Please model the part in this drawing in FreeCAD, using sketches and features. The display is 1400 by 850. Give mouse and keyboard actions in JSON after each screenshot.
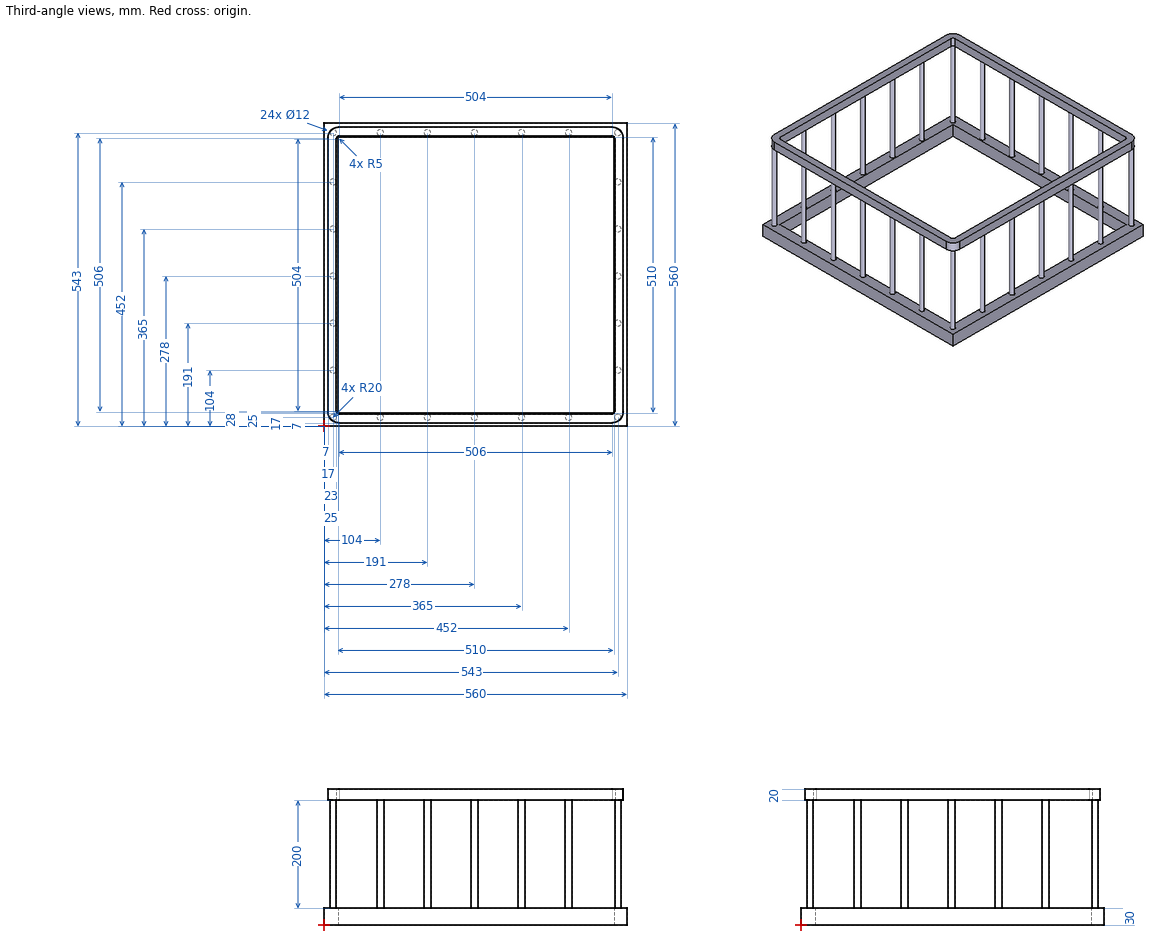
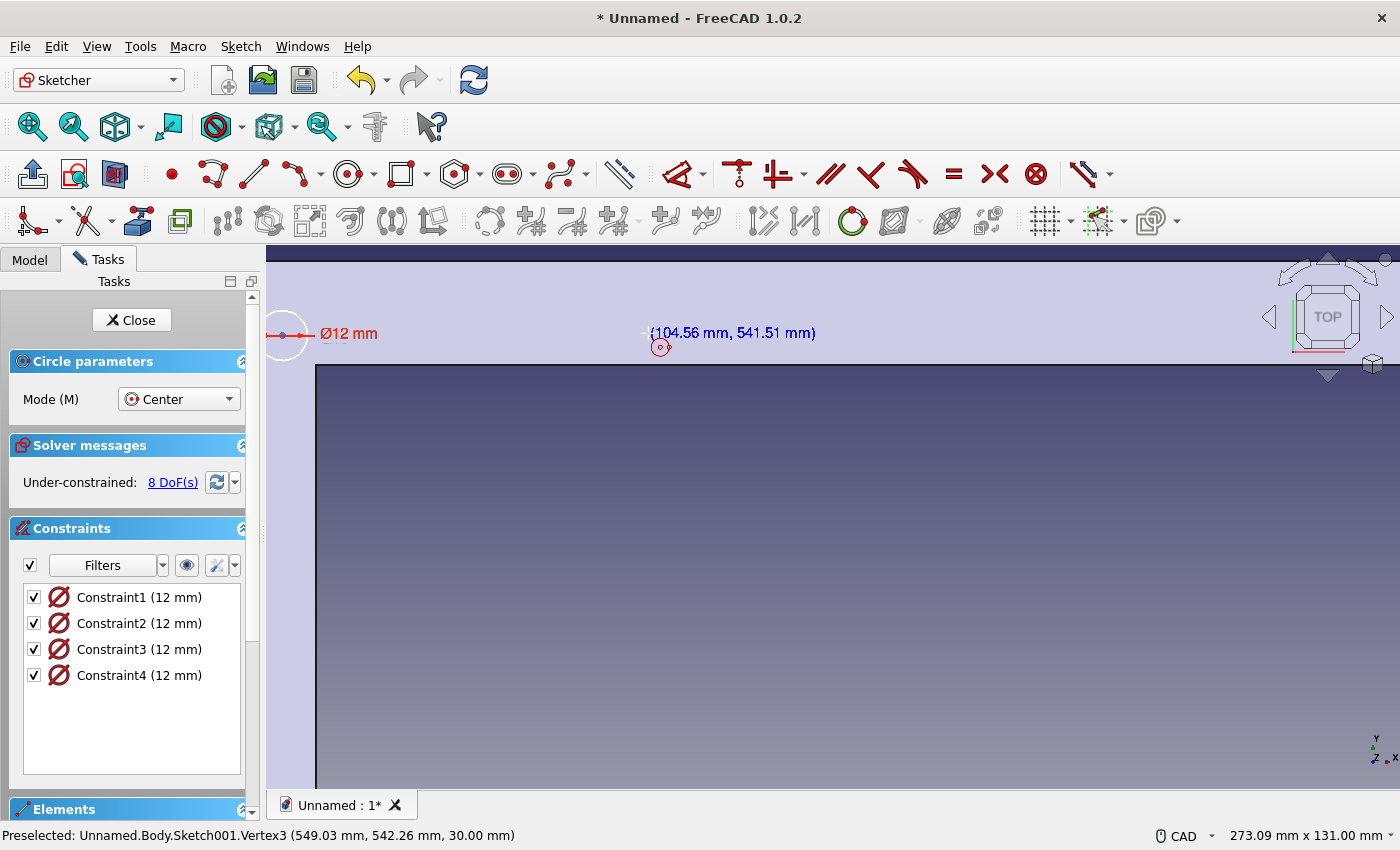
{"action": "scroll", "coordinate": [648, 333], "scroll_direction": "down", "scroll_amount": 9}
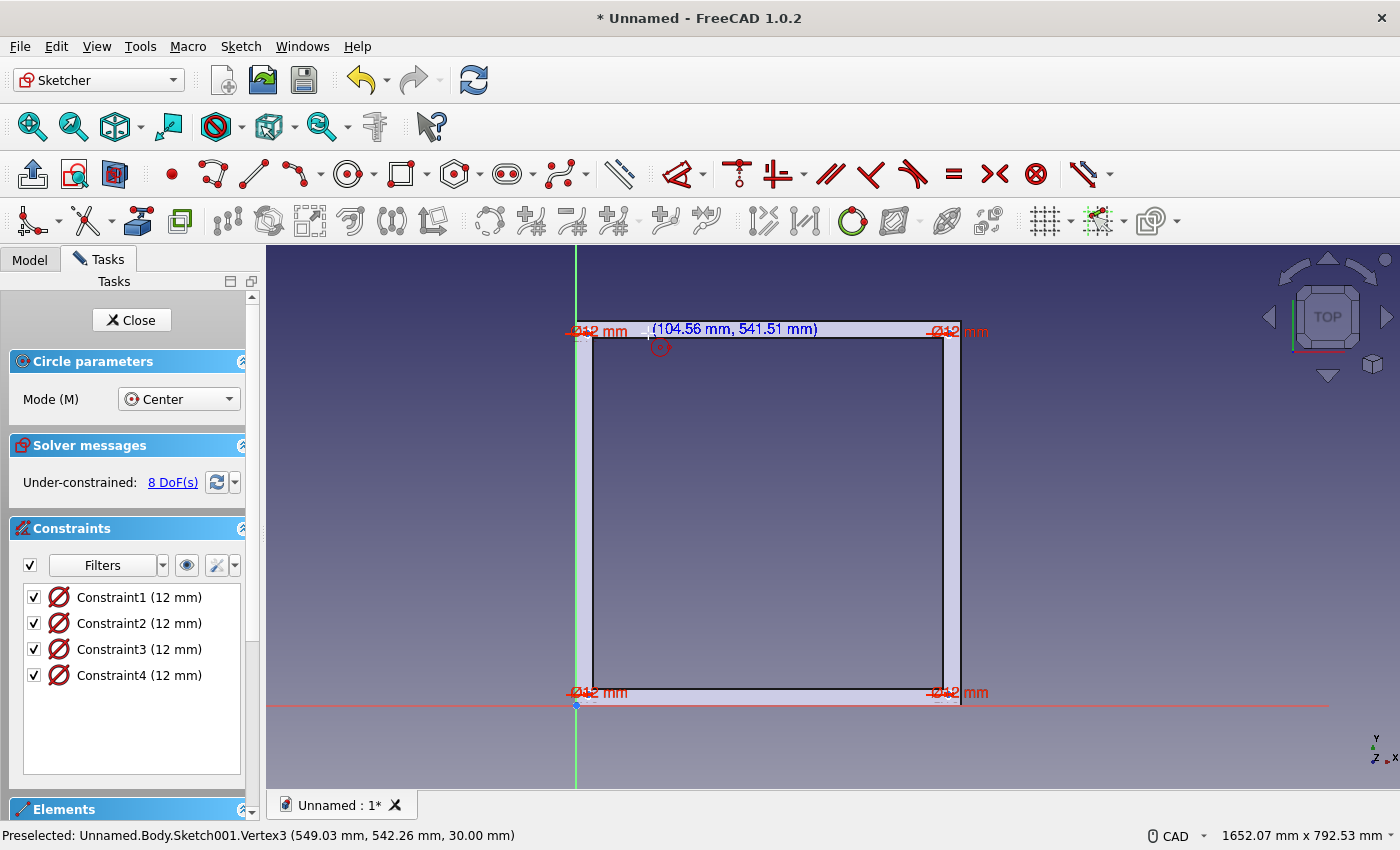
{"action": "left_click", "coordinate": [648, 333]}
{"action": "mouse_move", "coordinate": [651, 330]}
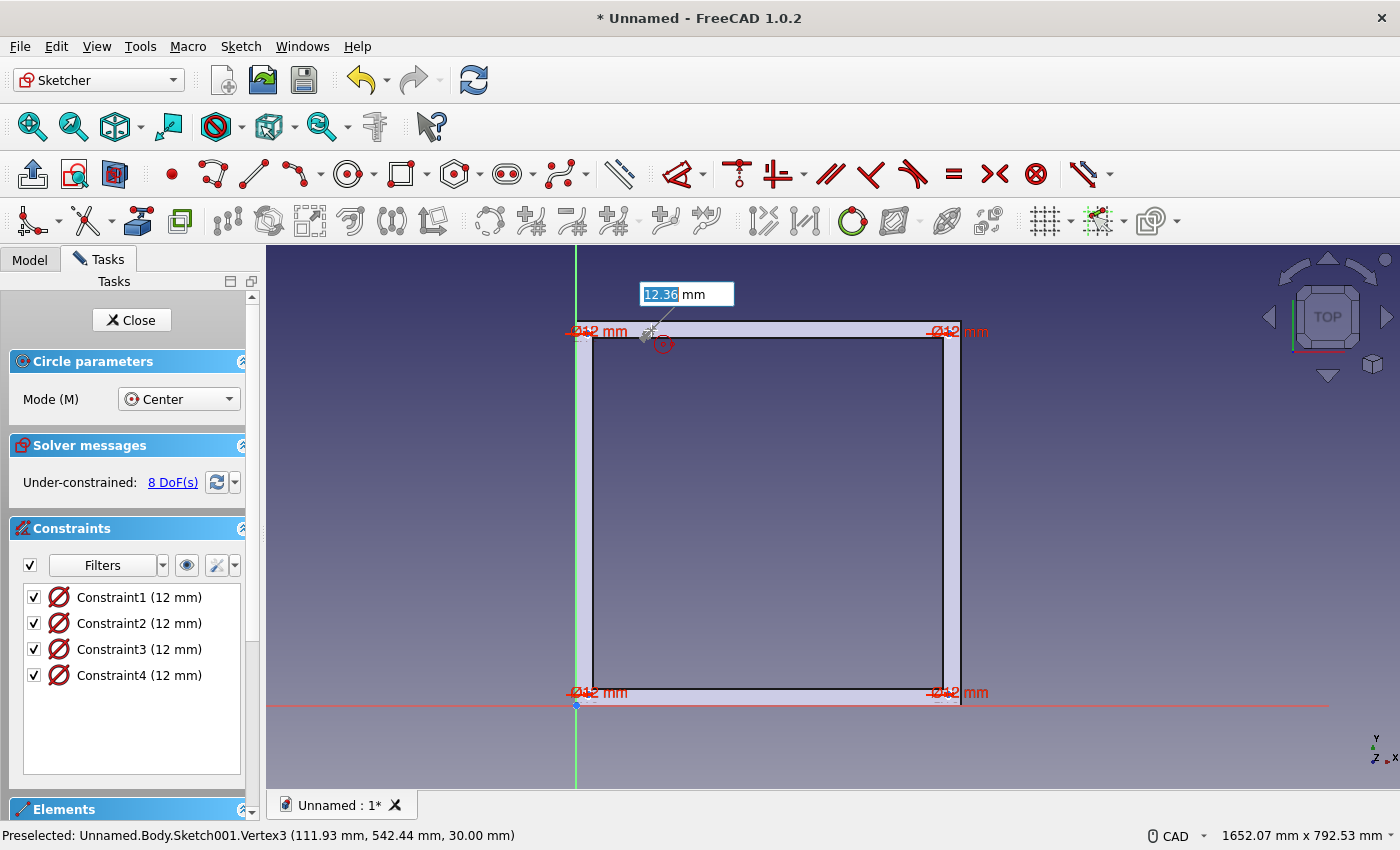
{"action": "type", "text": "12"}
{"action": "key", "text": "Return"}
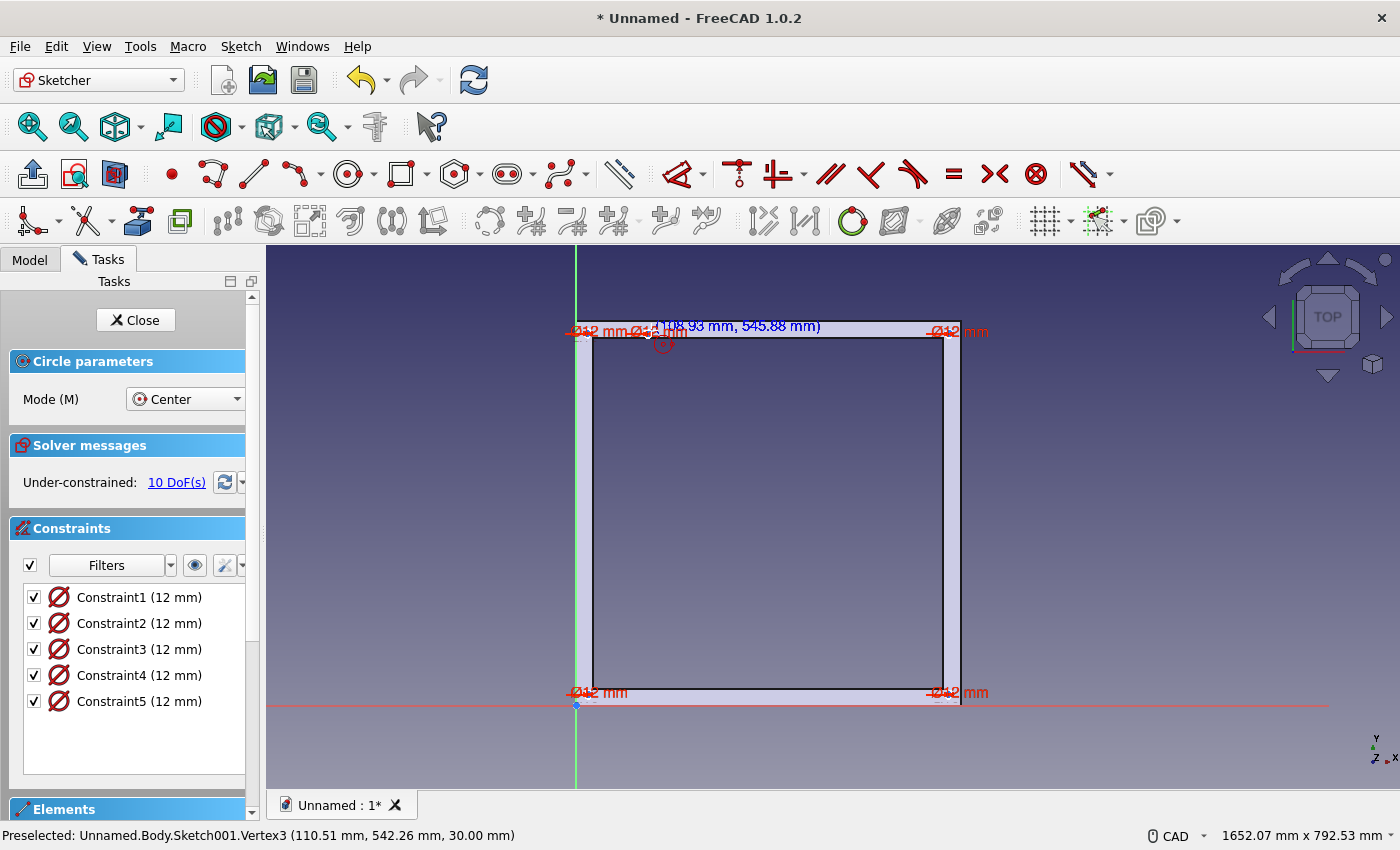
{"action": "scroll", "coordinate": [648, 694], "scroll_direction": "up", "scroll_amount": 9}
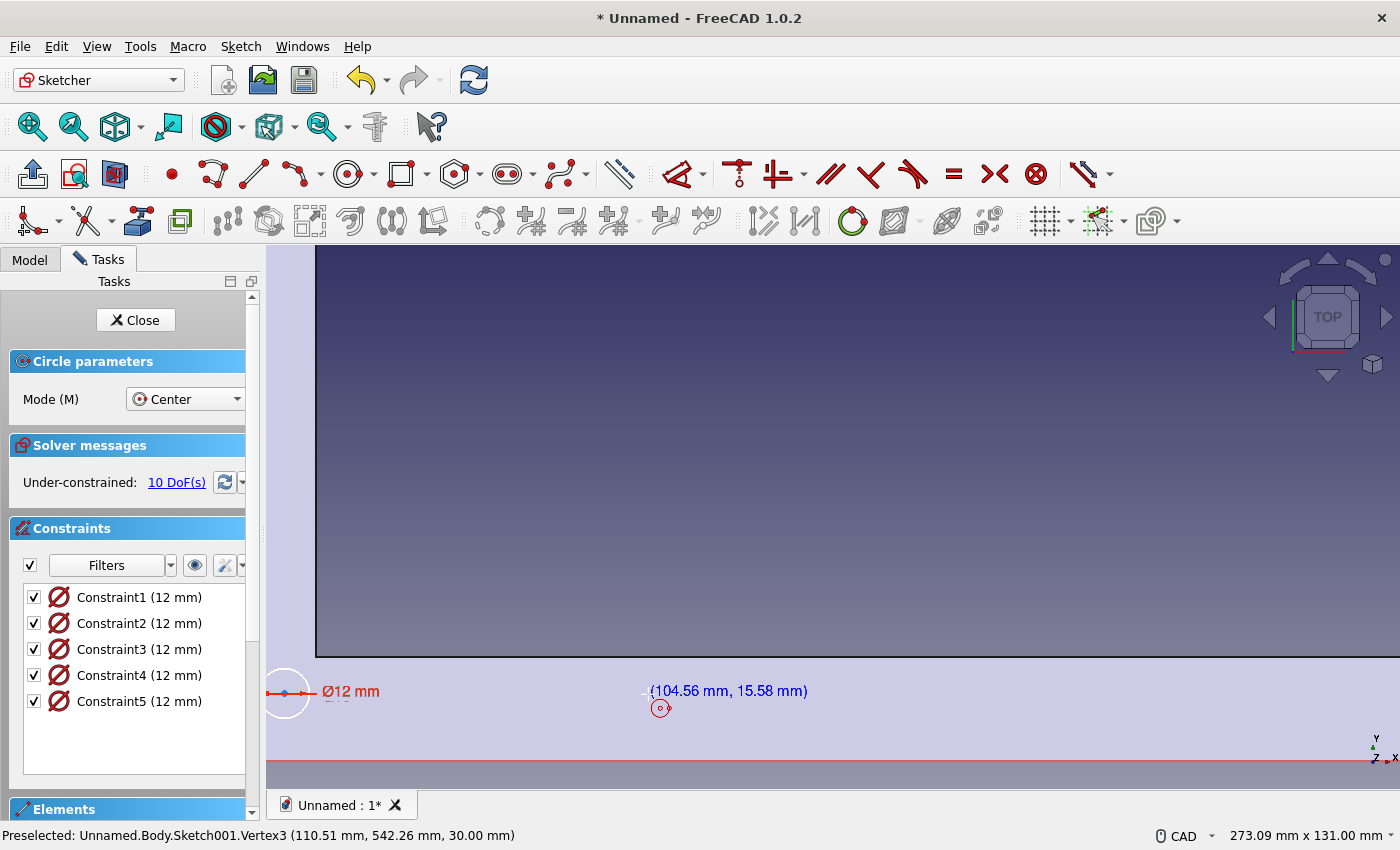
{"action": "scroll", "coordinate": [648, 694], "scroll_direction": "down", "scroll_amount": 9}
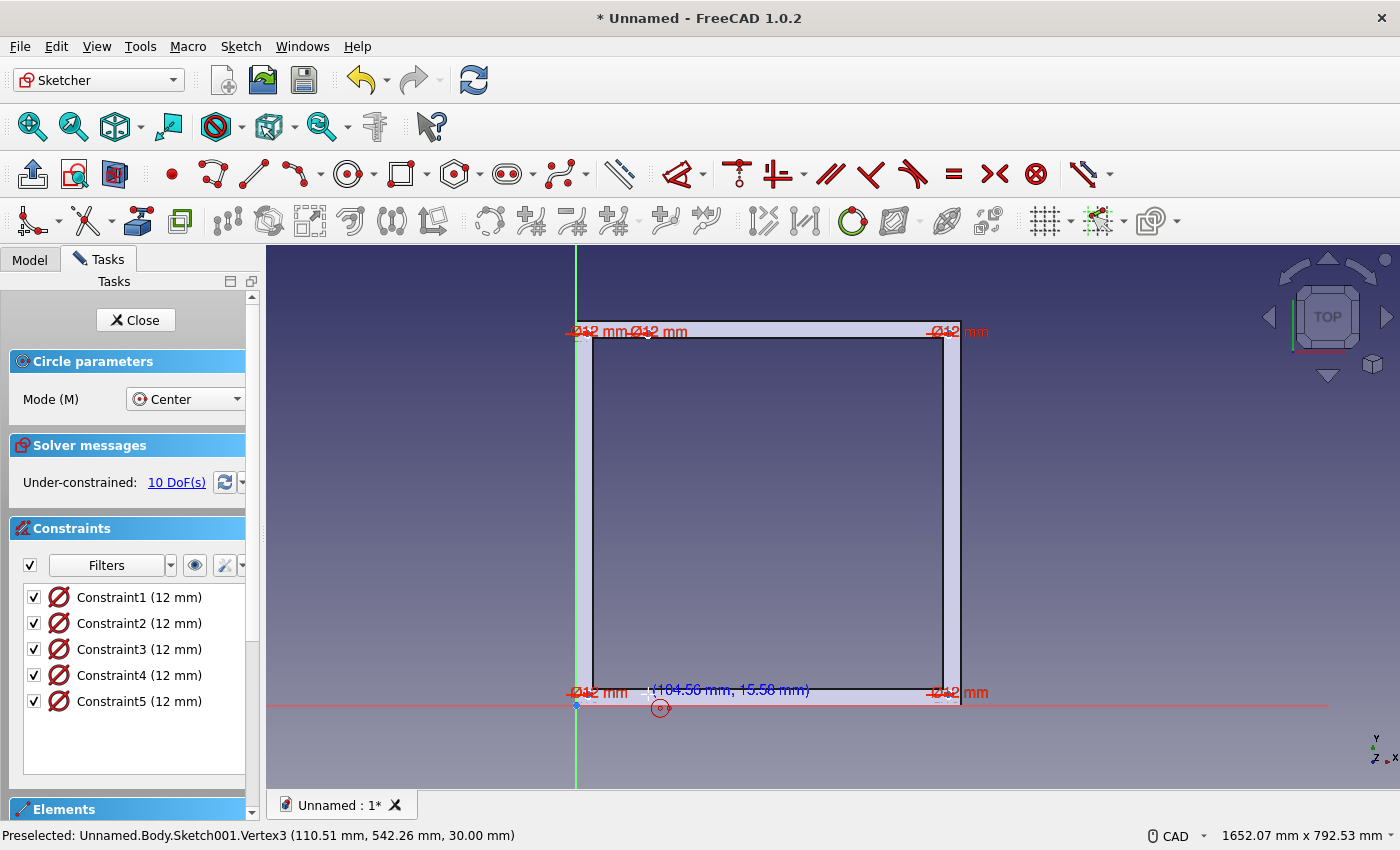
{"action": "scroll", "coordinate": [648, 694], "scroll_direction": "up", "scroll_amount": 2}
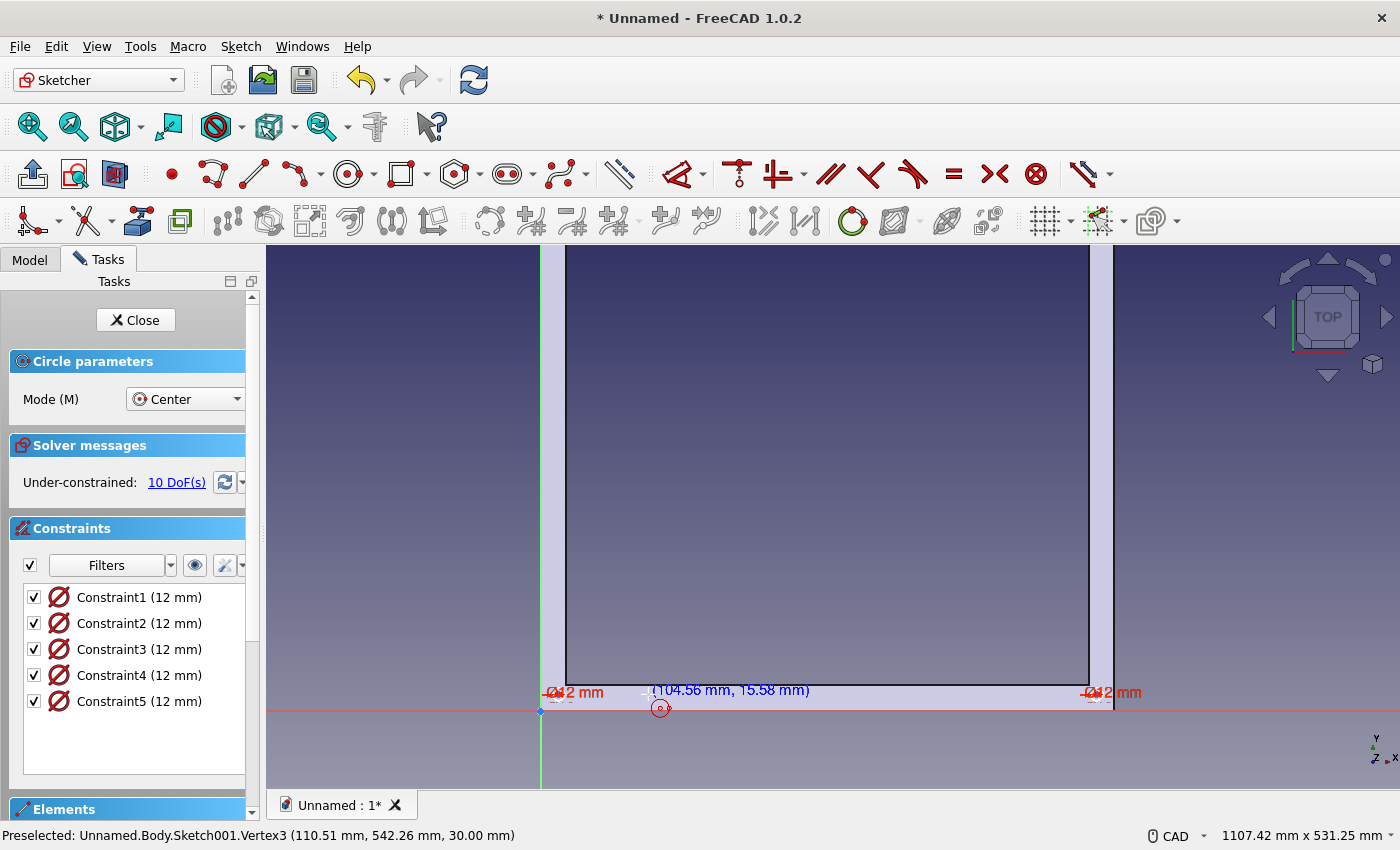
{"action": "left_click", "coordinate": [647, 694]}
{"action": "mouse_move", "coordinate": [652, 689]}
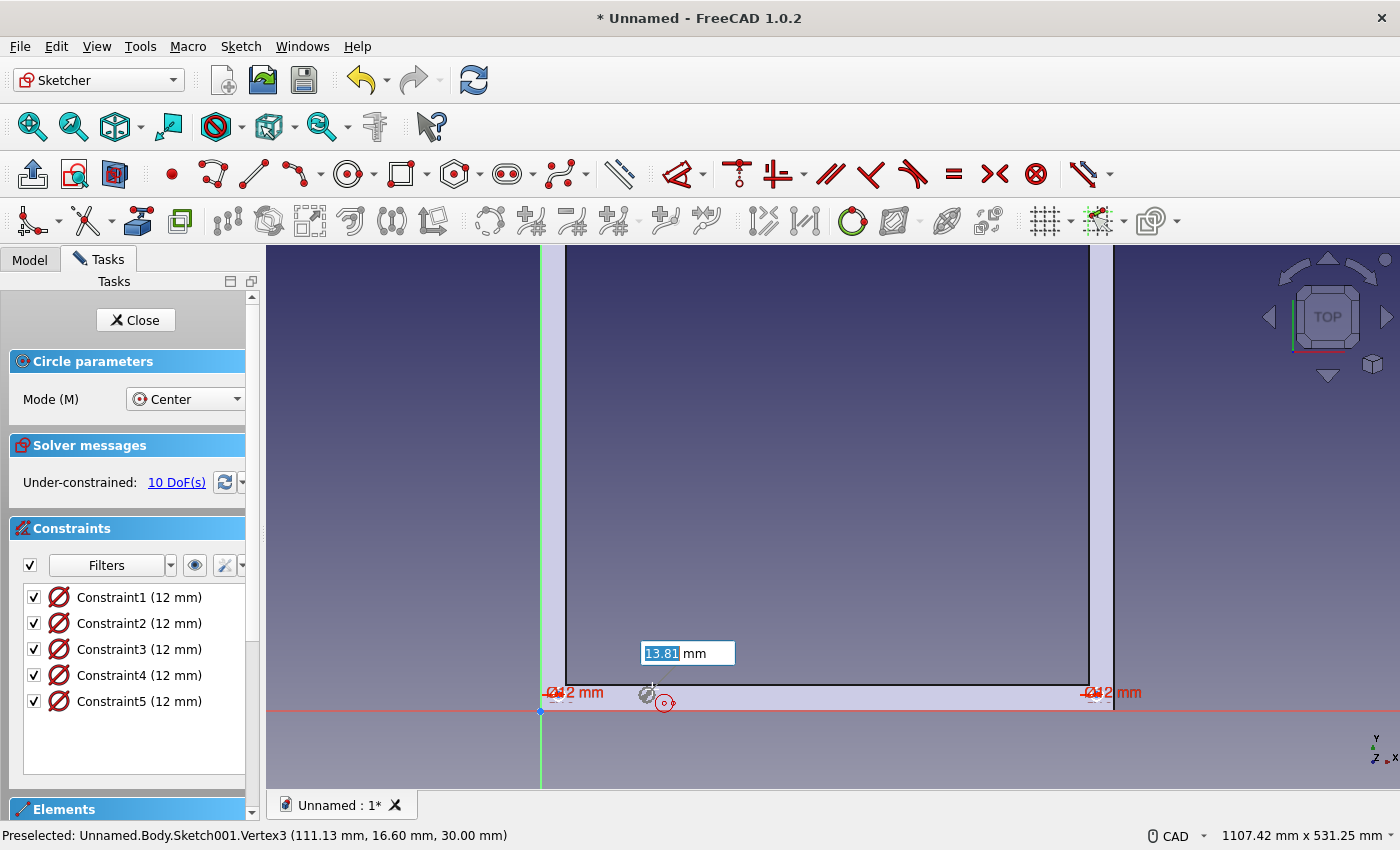
{"action": "type", "text": "12"}
{"action": "key", "text": "Return"}